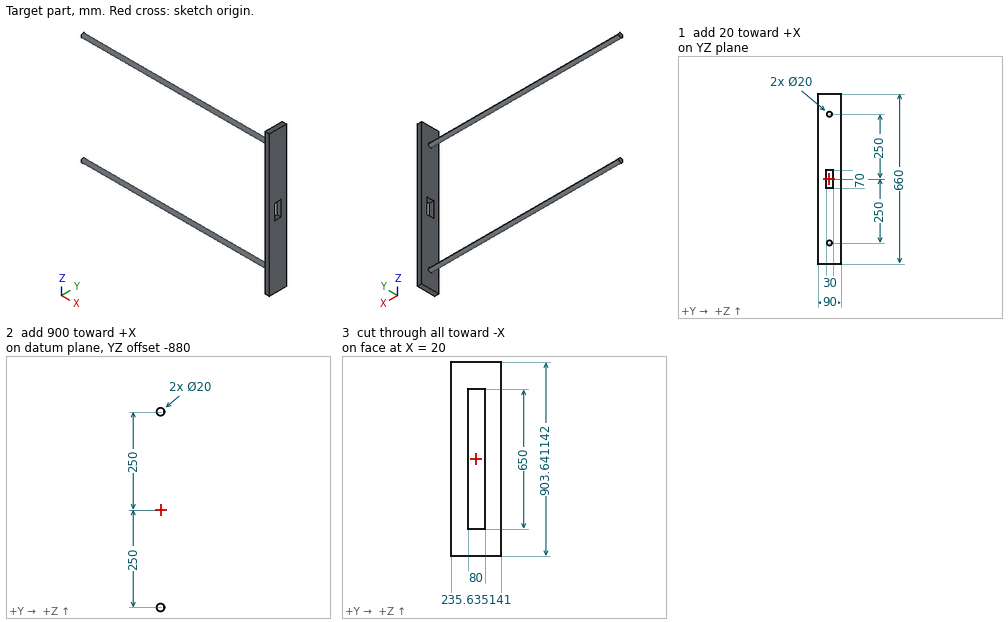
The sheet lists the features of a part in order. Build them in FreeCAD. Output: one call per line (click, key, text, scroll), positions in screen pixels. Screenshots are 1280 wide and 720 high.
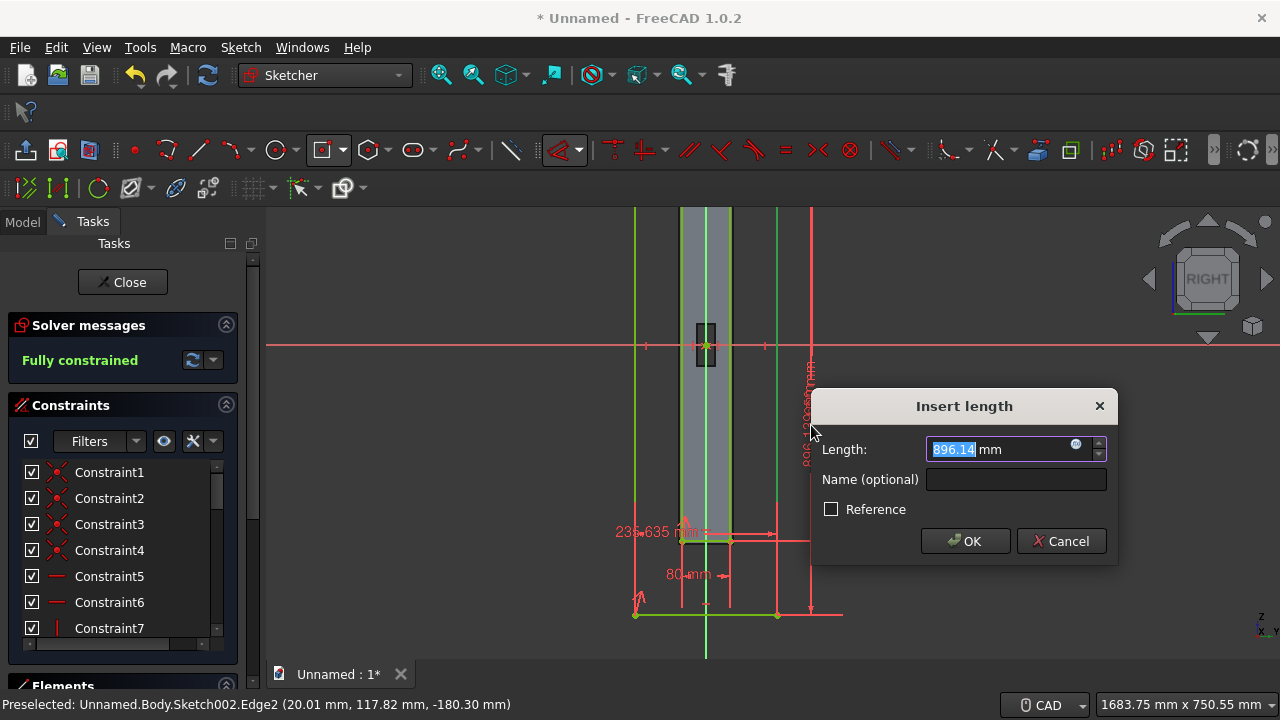
text(903.641142)
key(Return)
key(Escape)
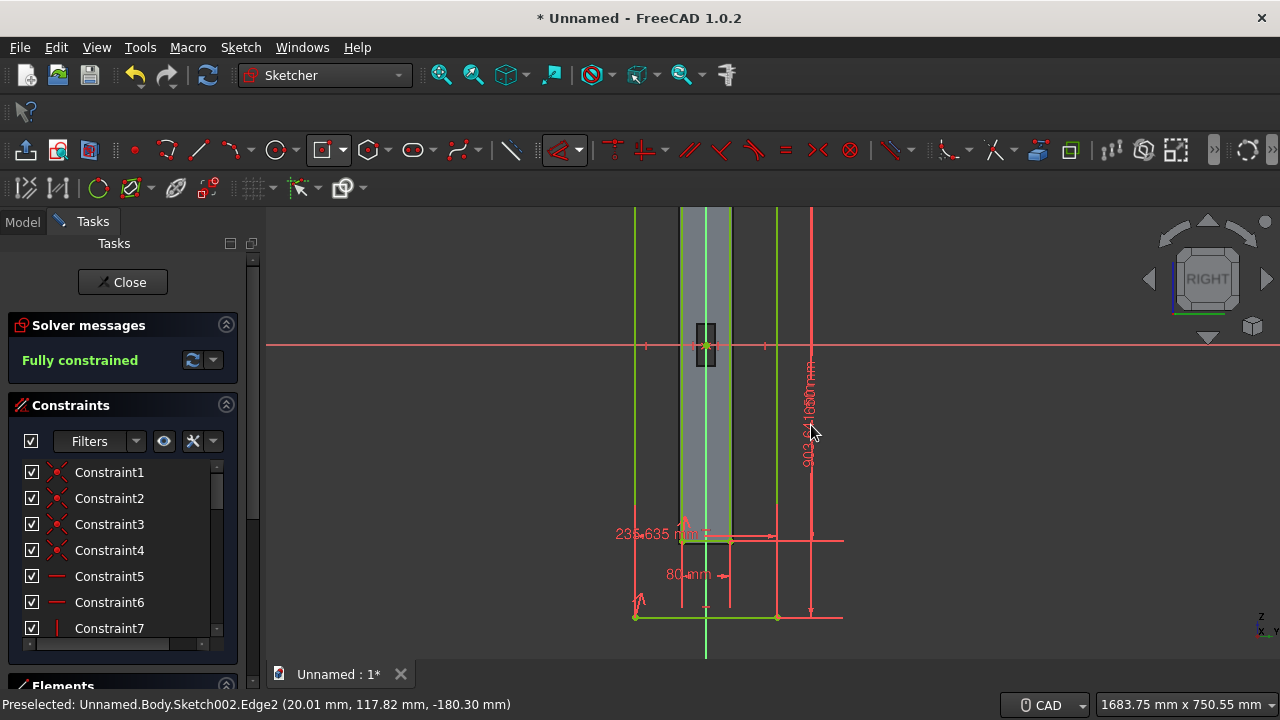
click(123, 282)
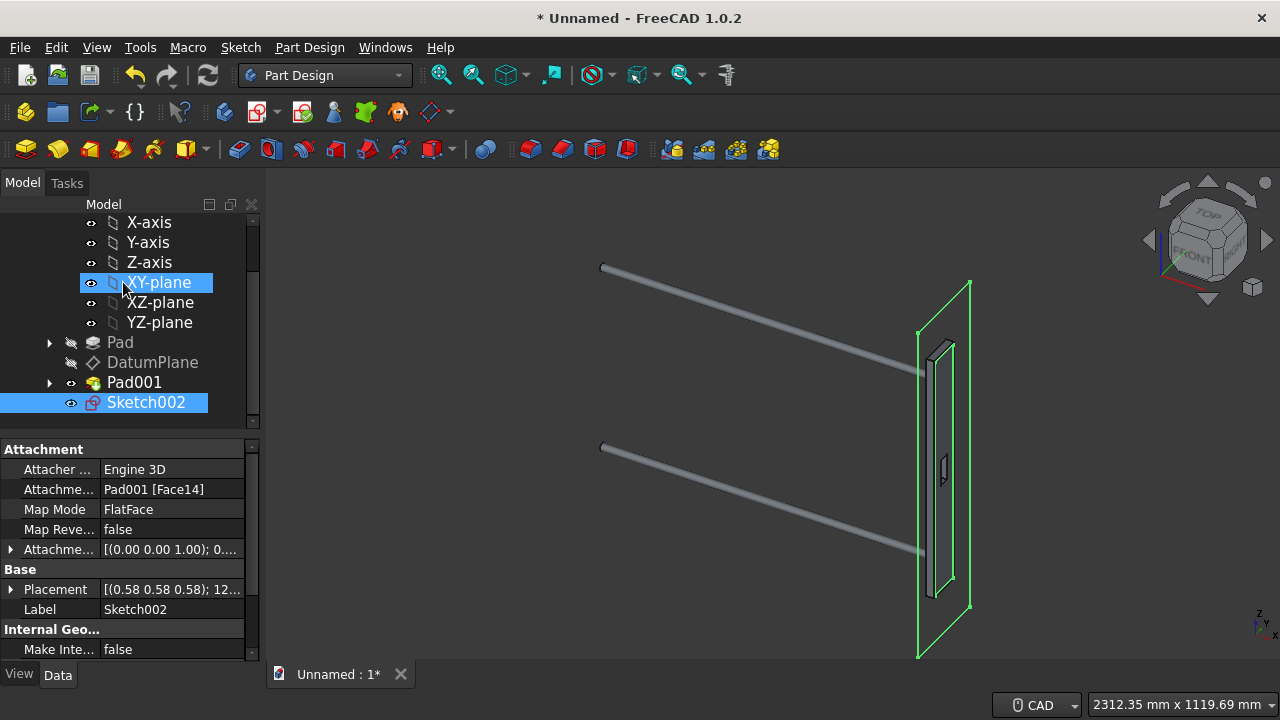
click(240, 150)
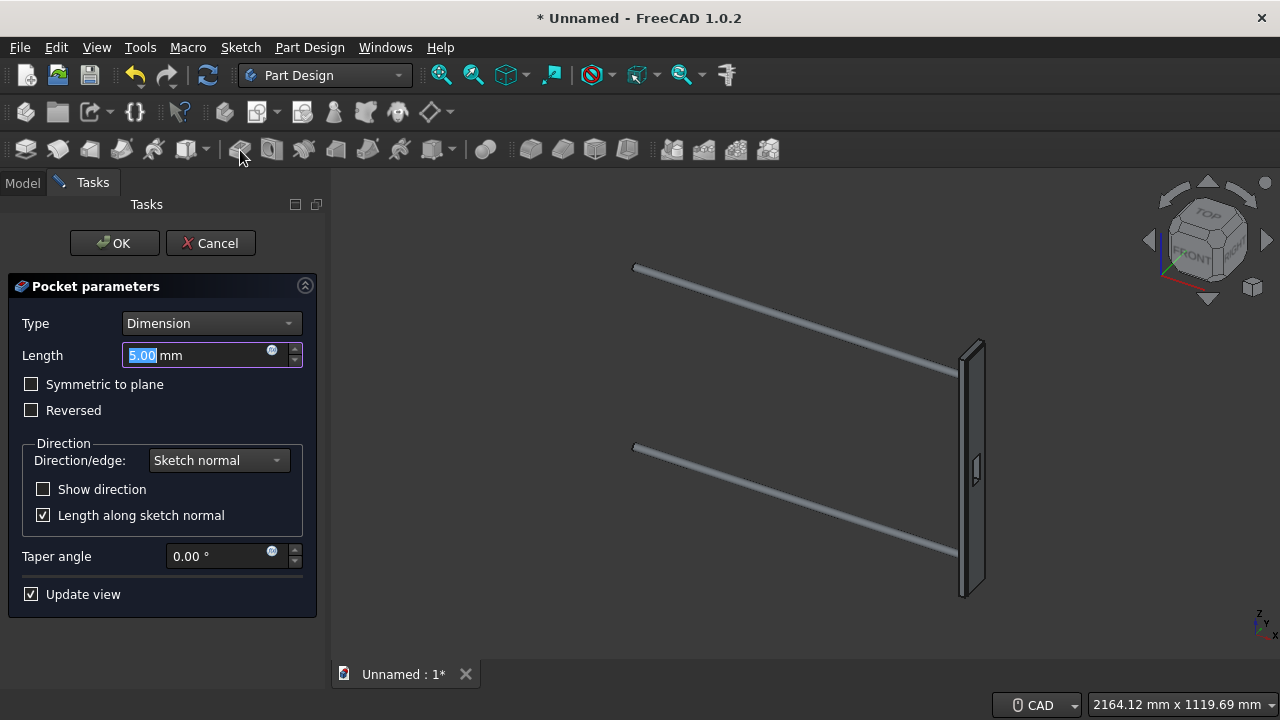
click(212, 324)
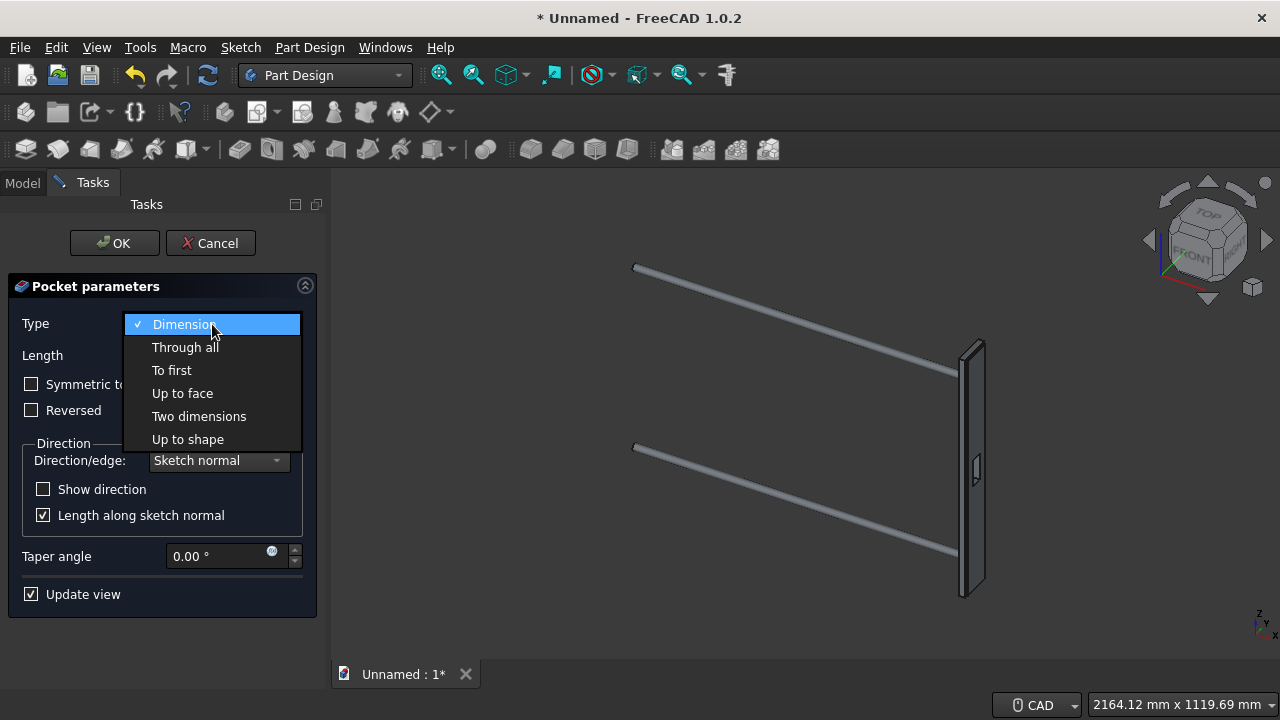
click(212, 348)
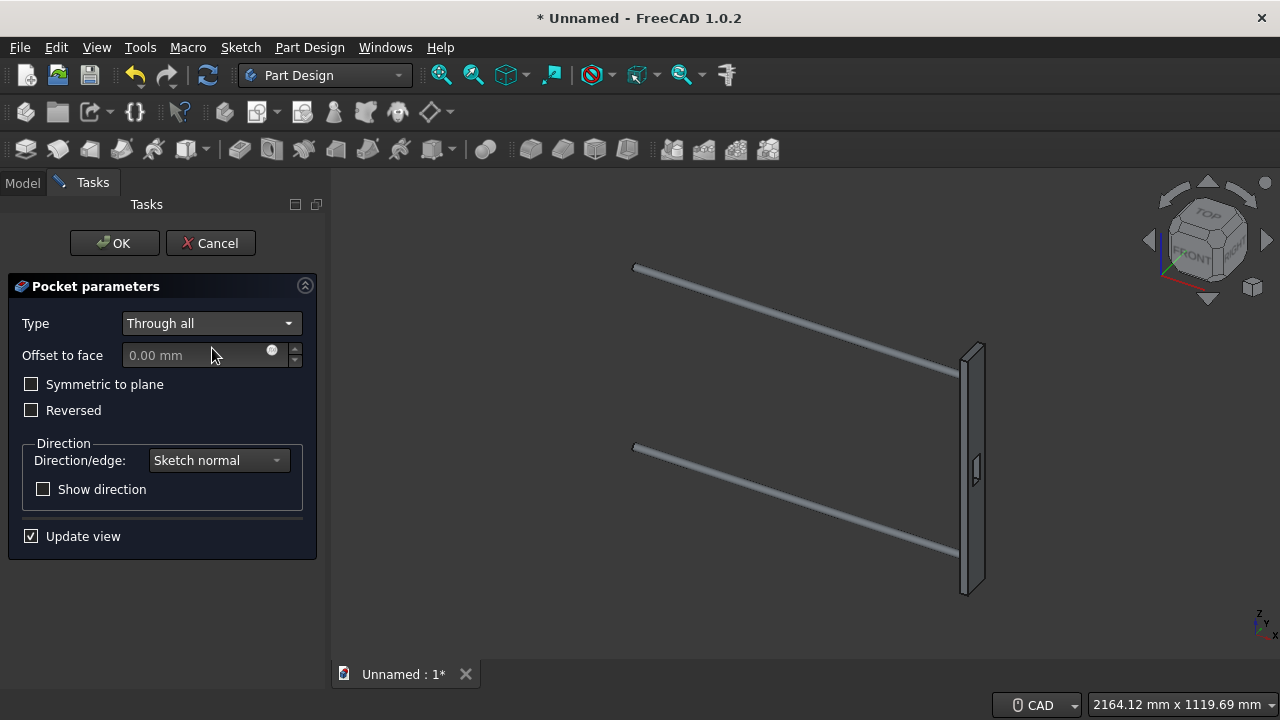
click(115, 243)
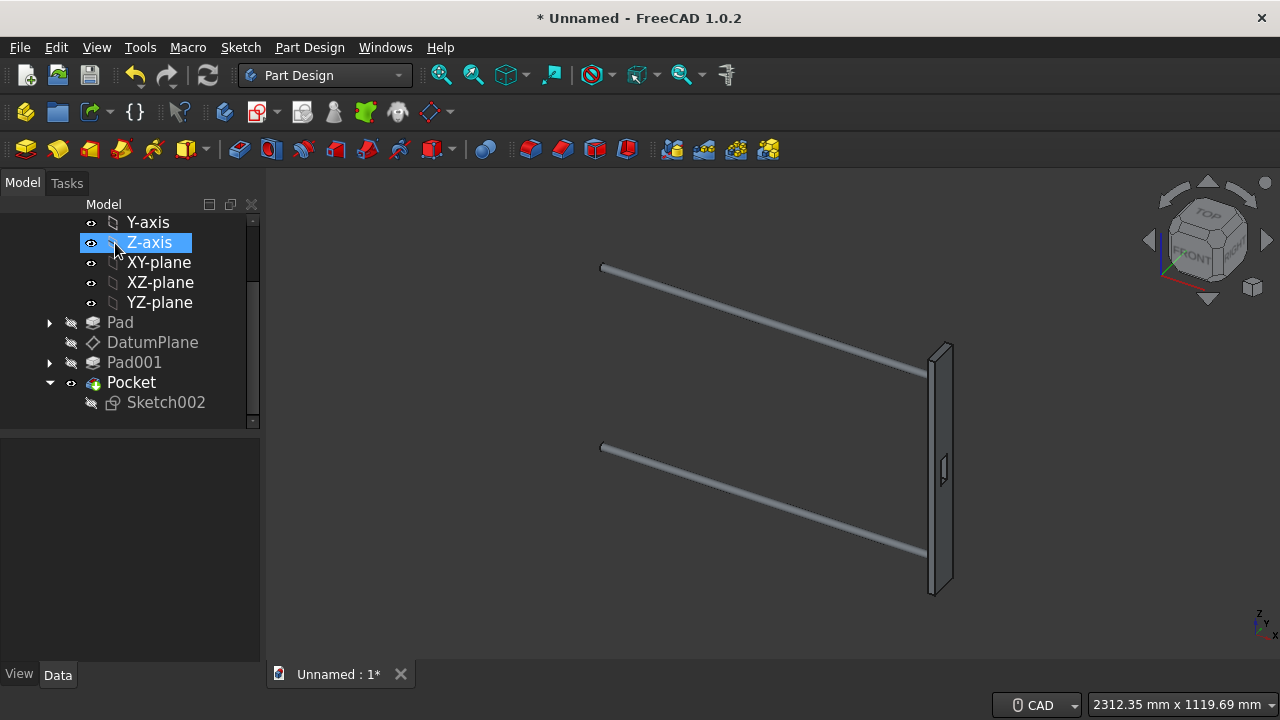
key(0)